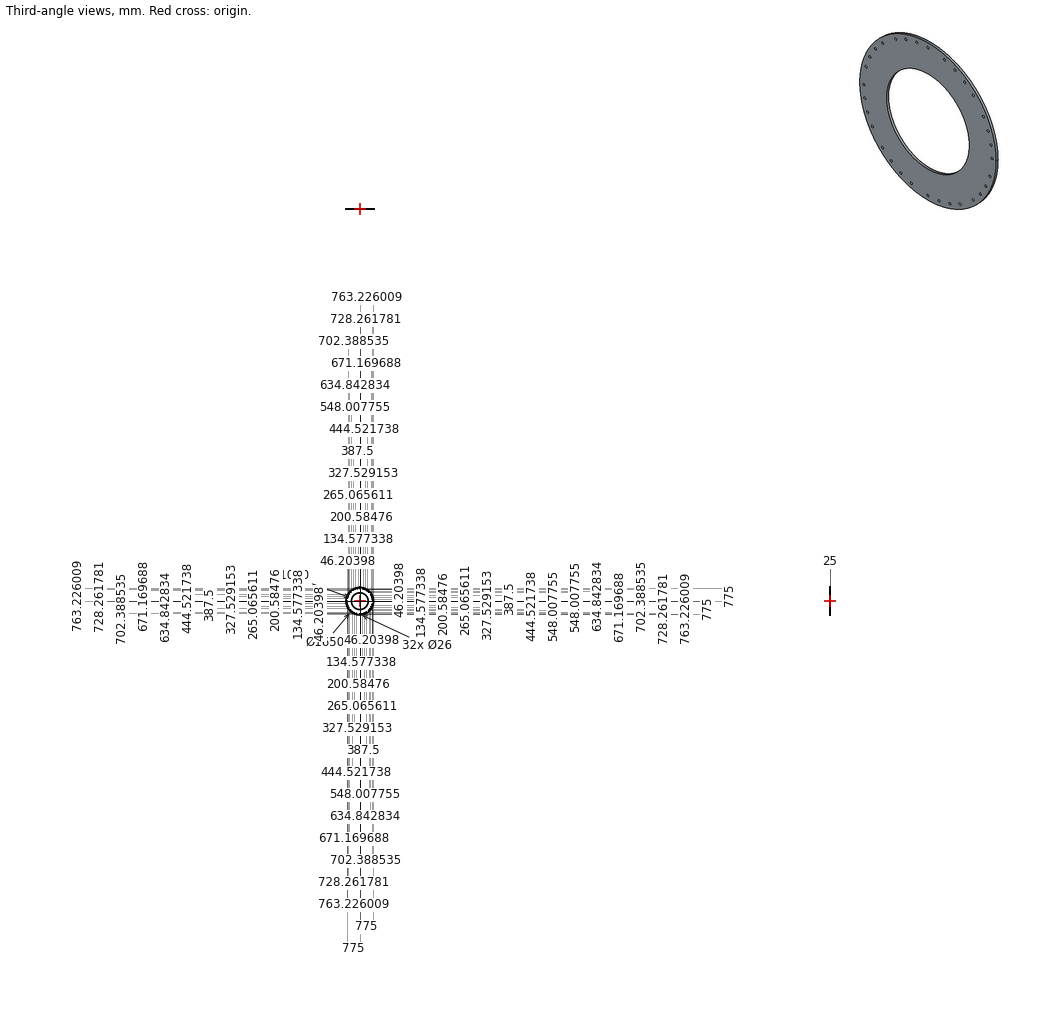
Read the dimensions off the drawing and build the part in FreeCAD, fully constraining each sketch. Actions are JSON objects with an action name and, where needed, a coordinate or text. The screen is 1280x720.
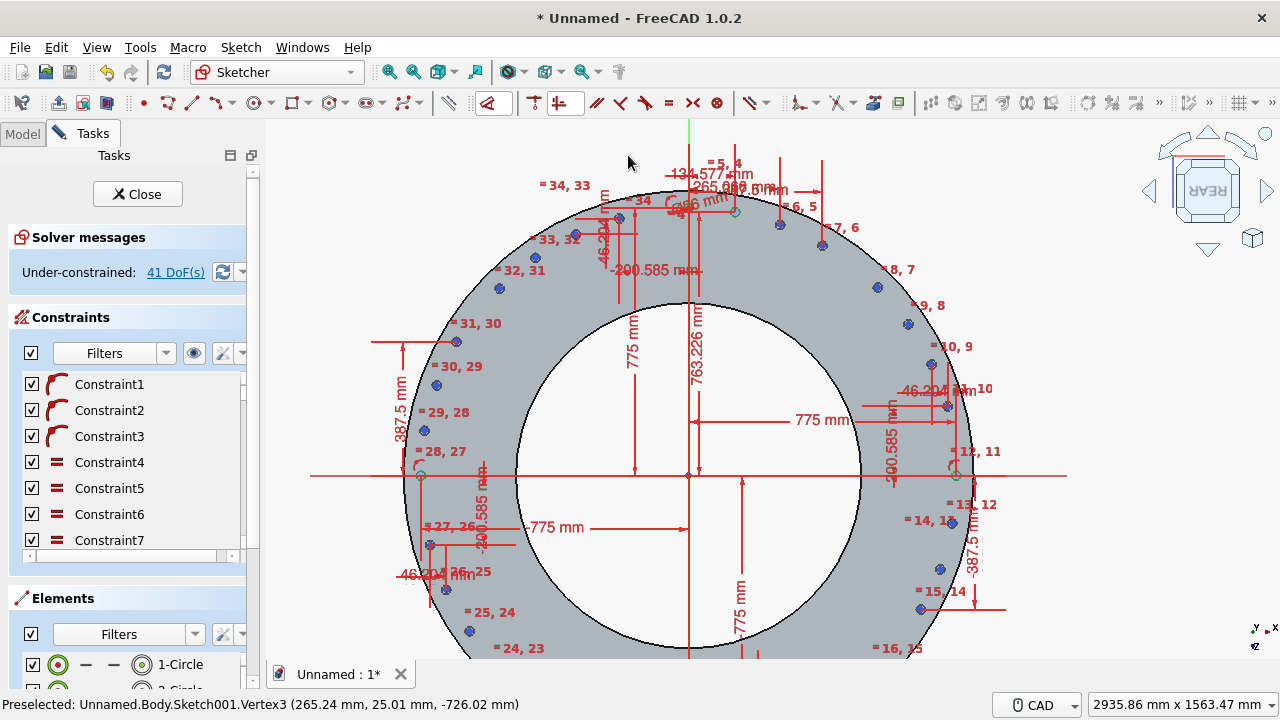
{"action": "left_click", "coordinate": [780, 225]}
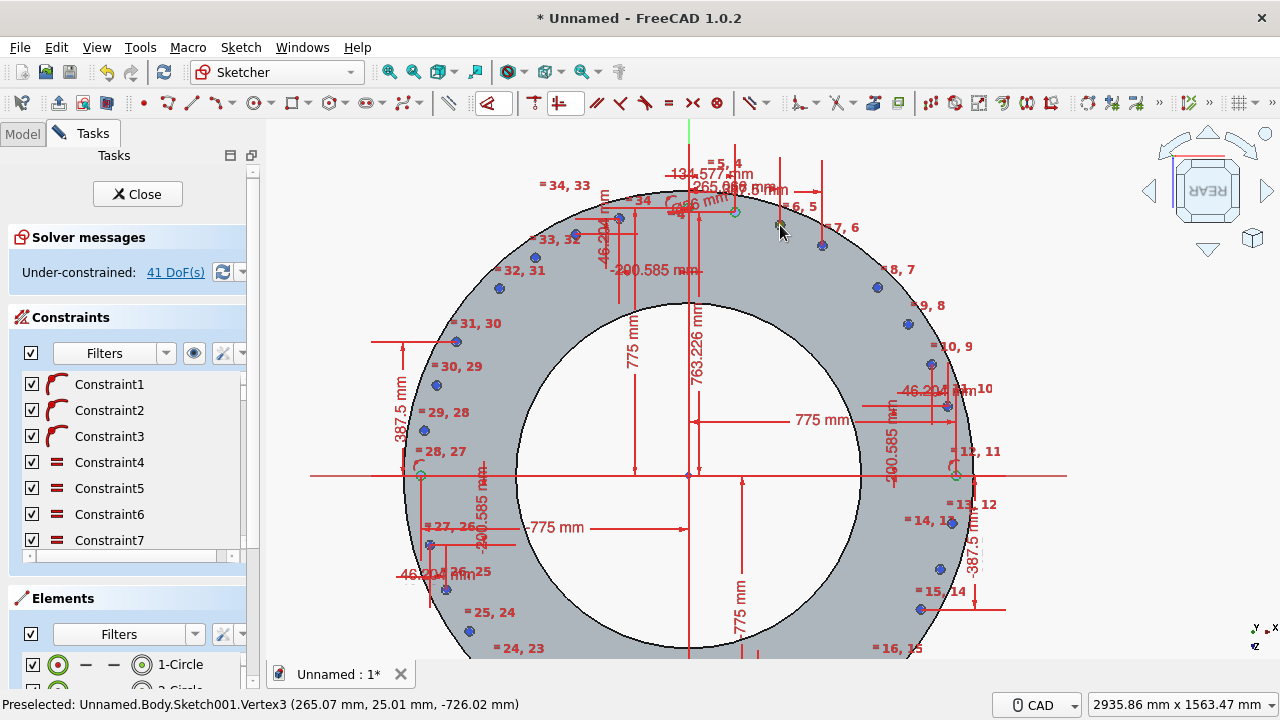
{"action": "key", "text": "i"}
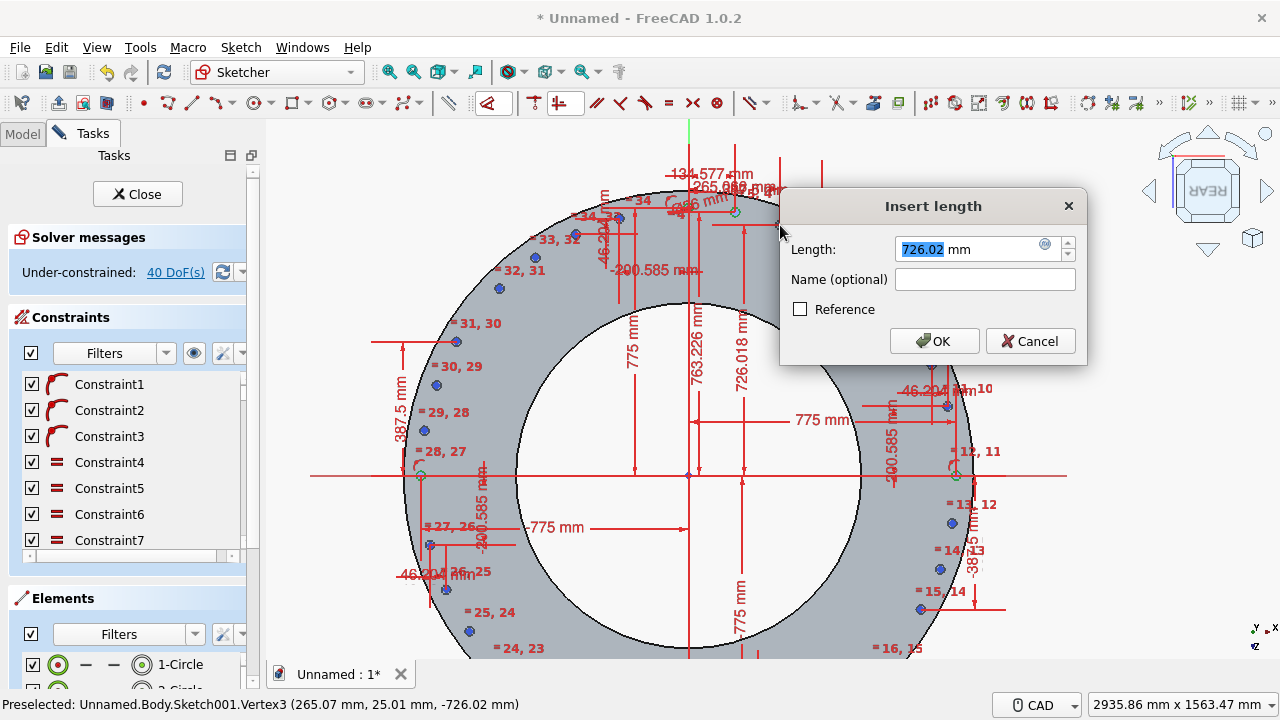
{"action": "type", "text": "728.261781"}
{"action": "key", "text": "Return"}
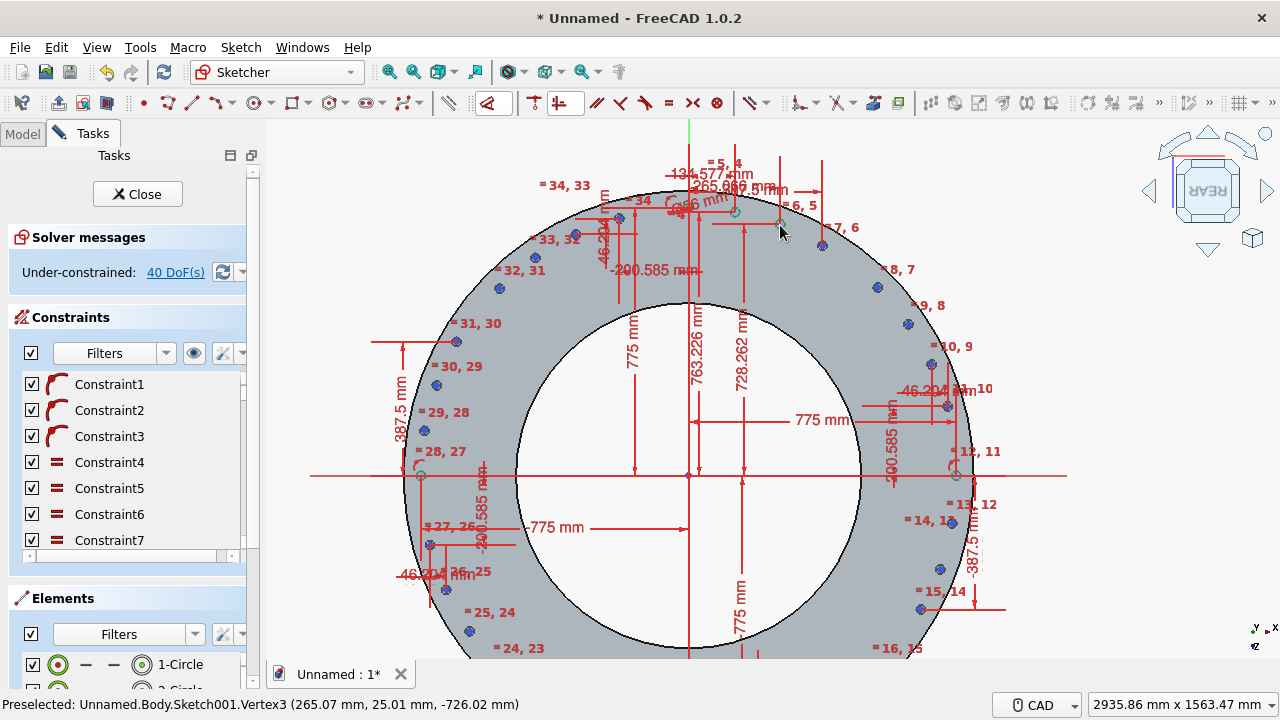
{"action": "left_click", "coordinate": [822, 246]}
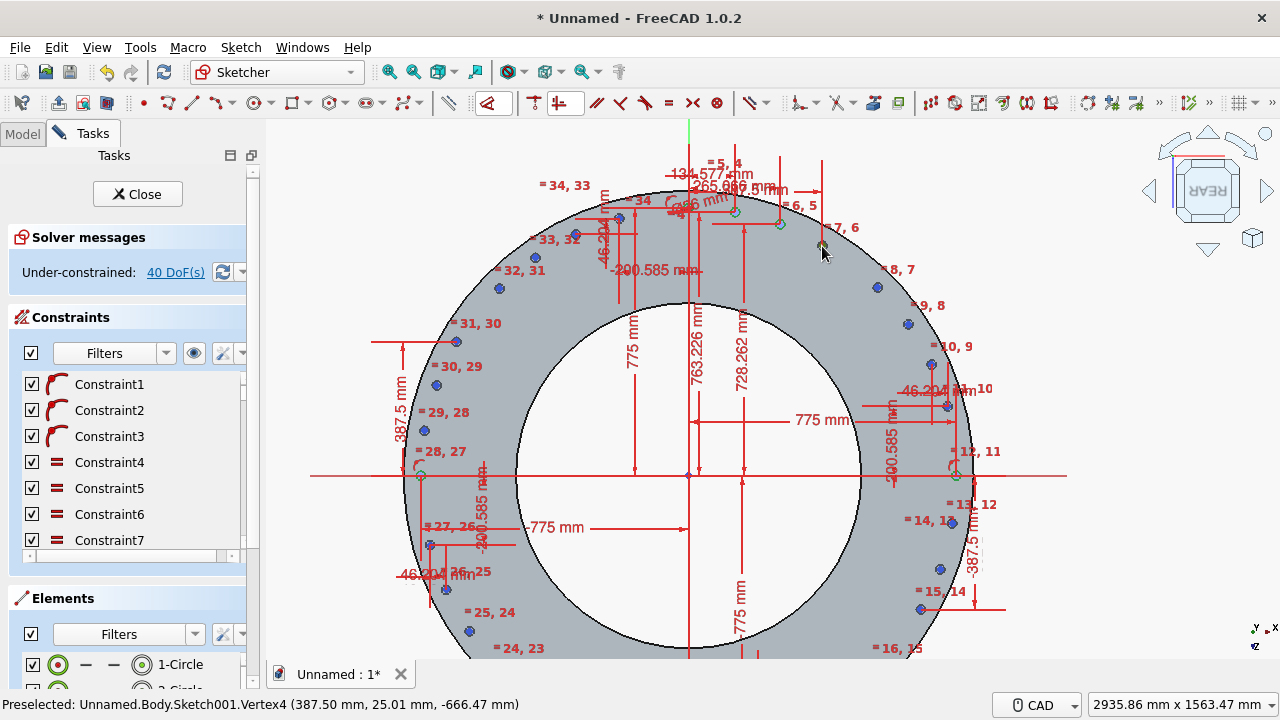
{"action": "key", "text": "i"}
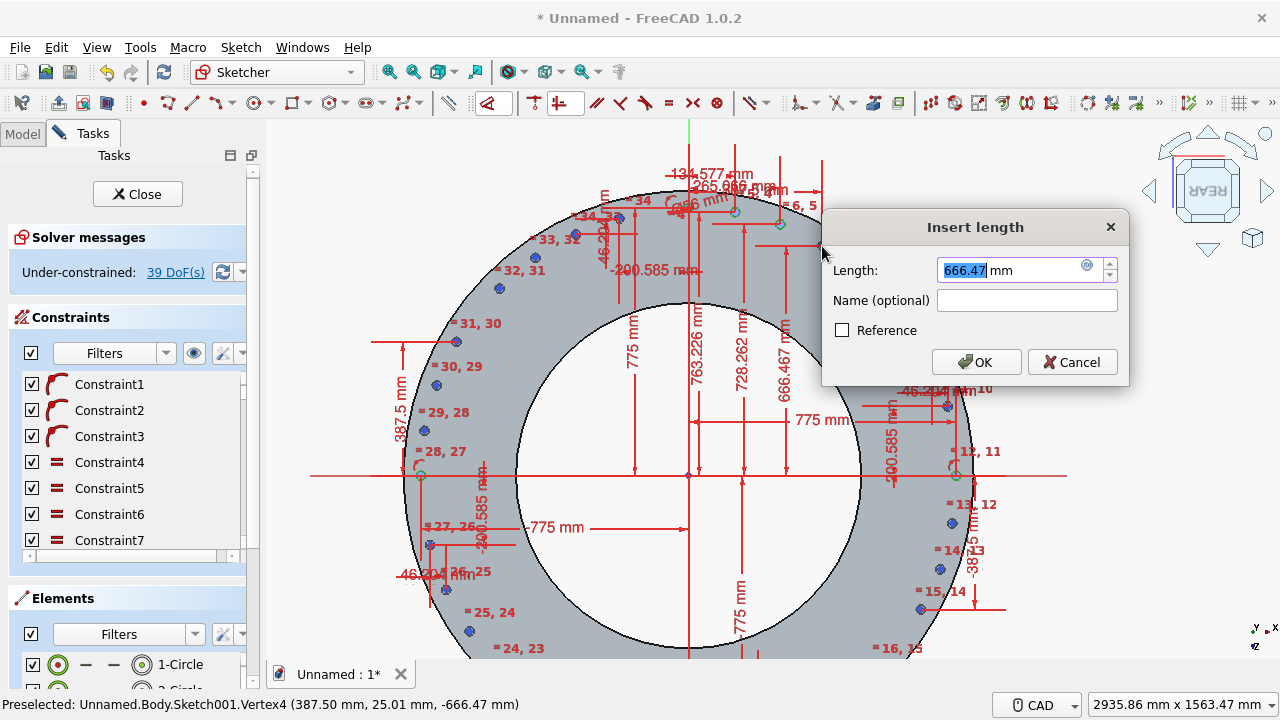
{"action": "type", "text": "671.169688"}
{"action": "key", "text": "Return"}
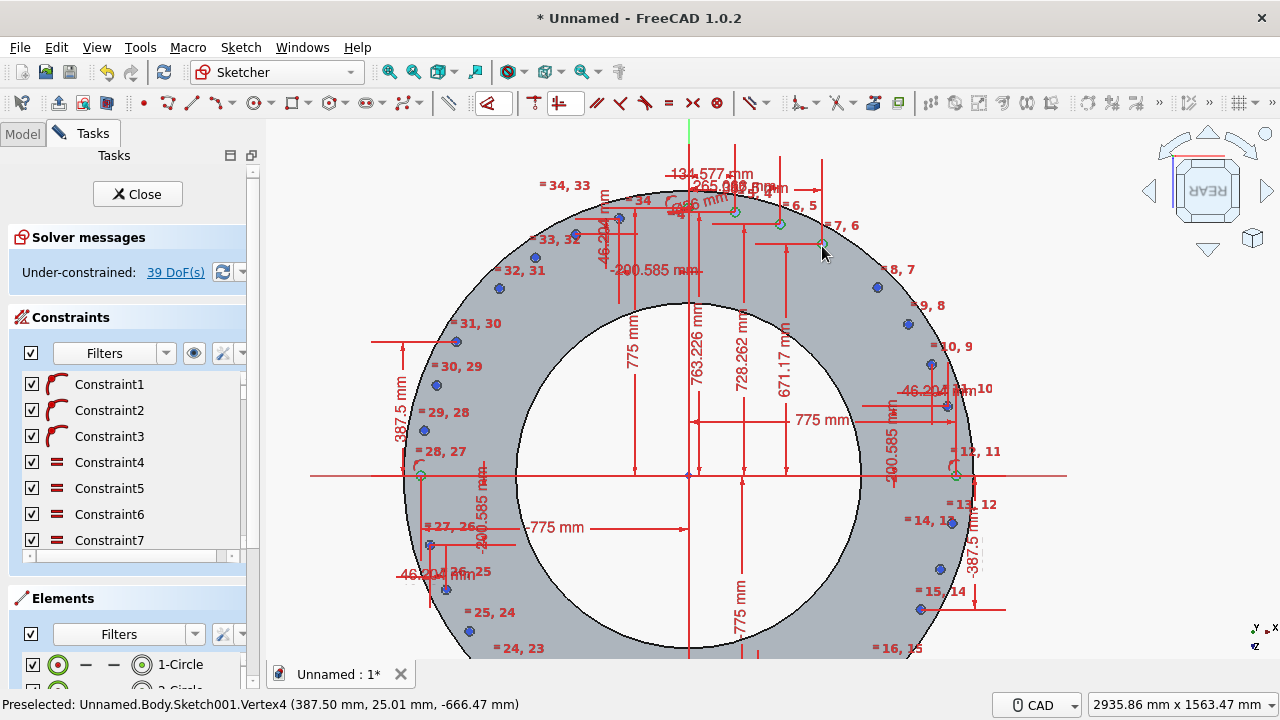
{"action": "left_click", "coordinate": [878, 288]}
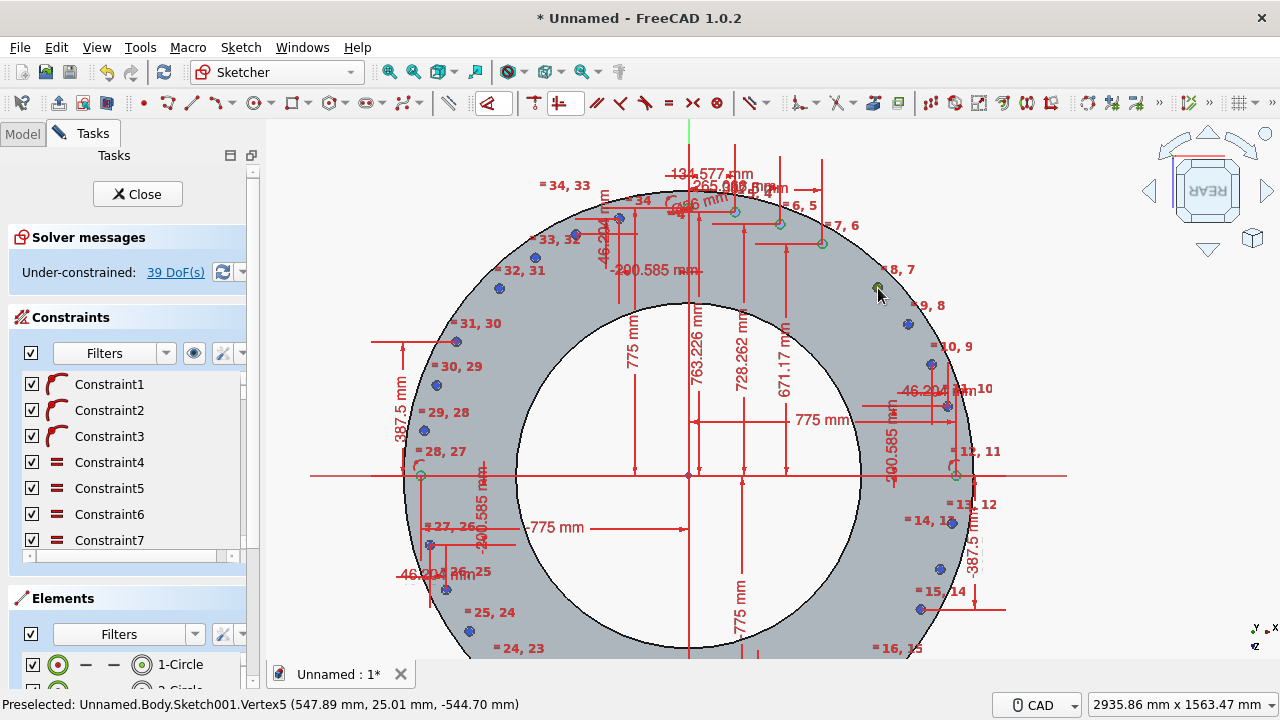
{"action": "key", "text": "l"}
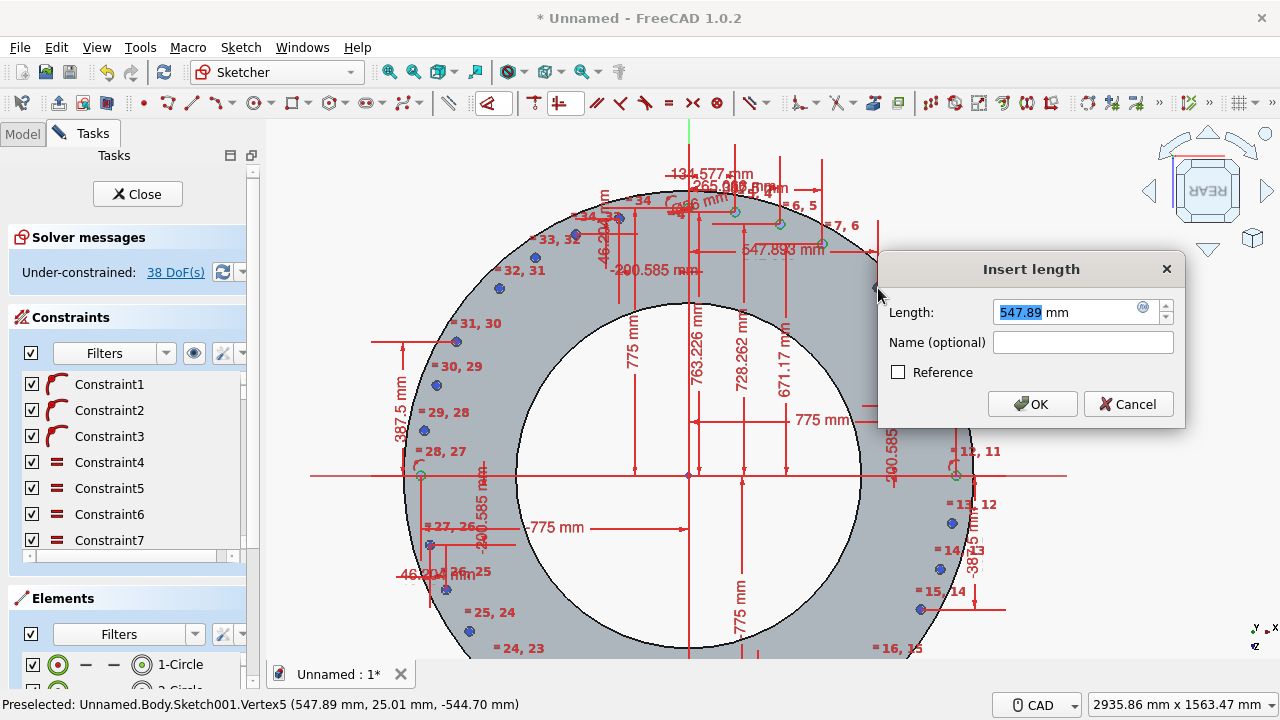
{"action": "type", "text": "548.007755"}
{"action": "key", "text": "Return"}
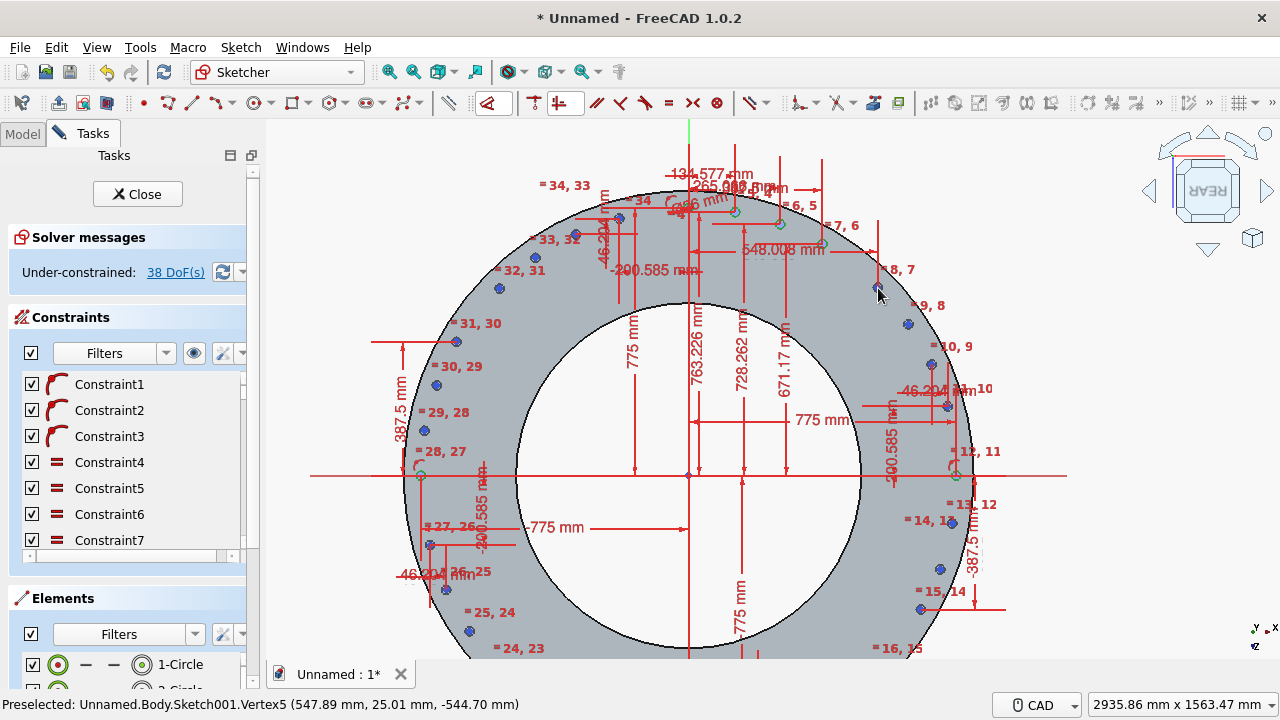
{"action": "left_click", "coordinate": [878, 288]}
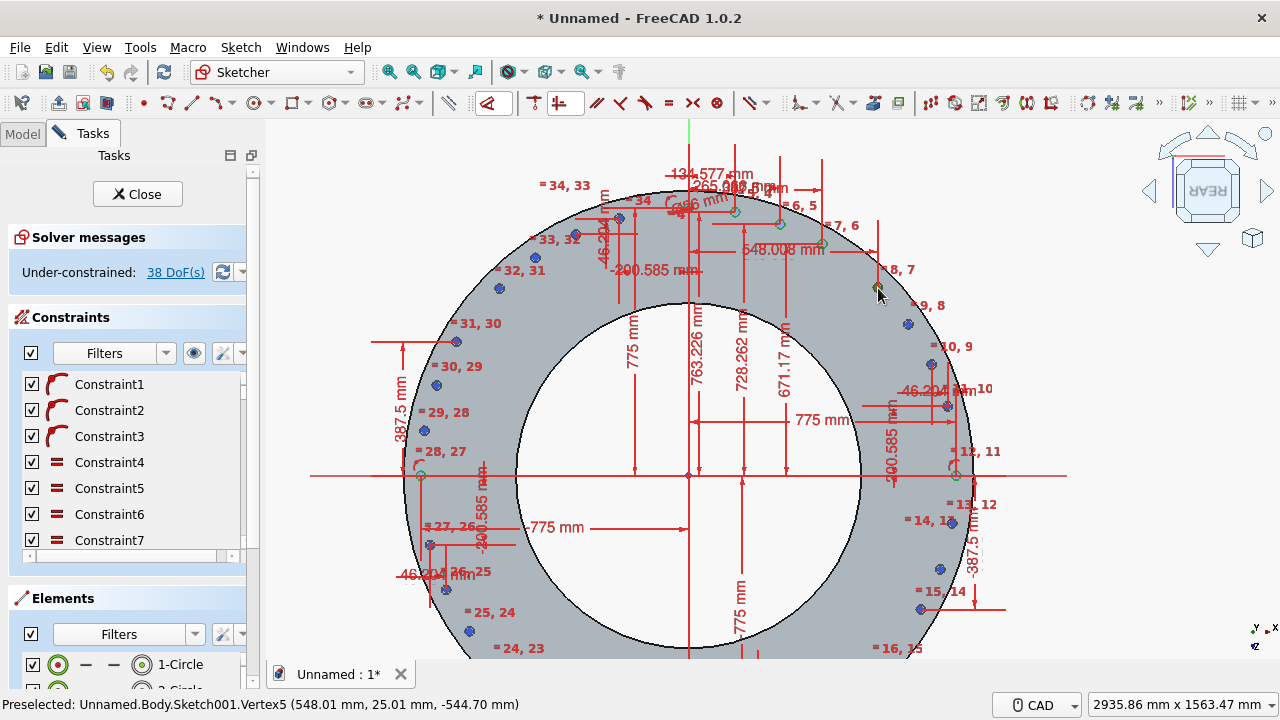
{"action": "key", "text": "i"}